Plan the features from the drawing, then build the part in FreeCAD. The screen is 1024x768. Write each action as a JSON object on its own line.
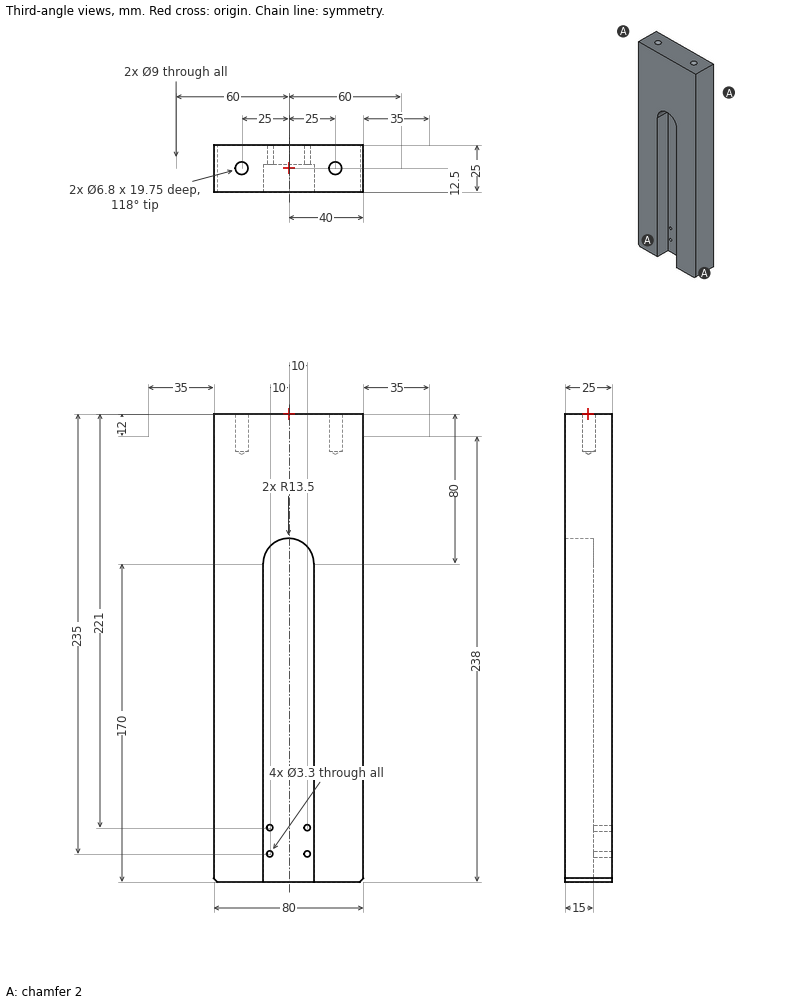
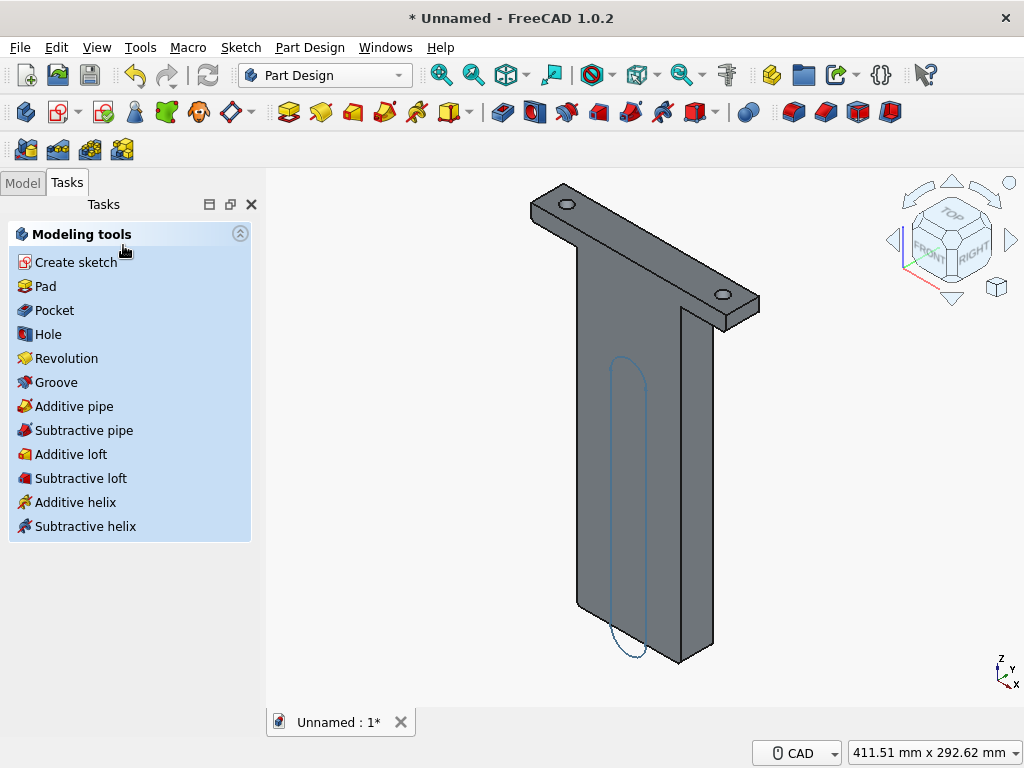
{"action": "left_click", "coordinate": [504, 112]}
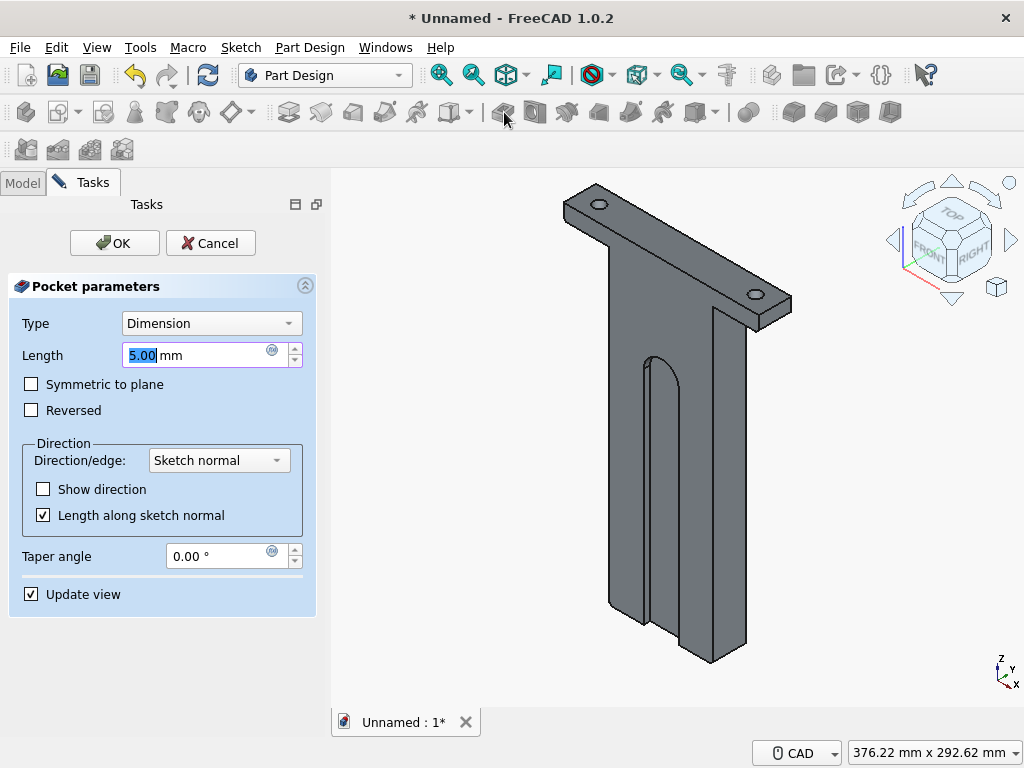
{"action": "type", "text": "15"}
{"action": "key", "text": "Tab"}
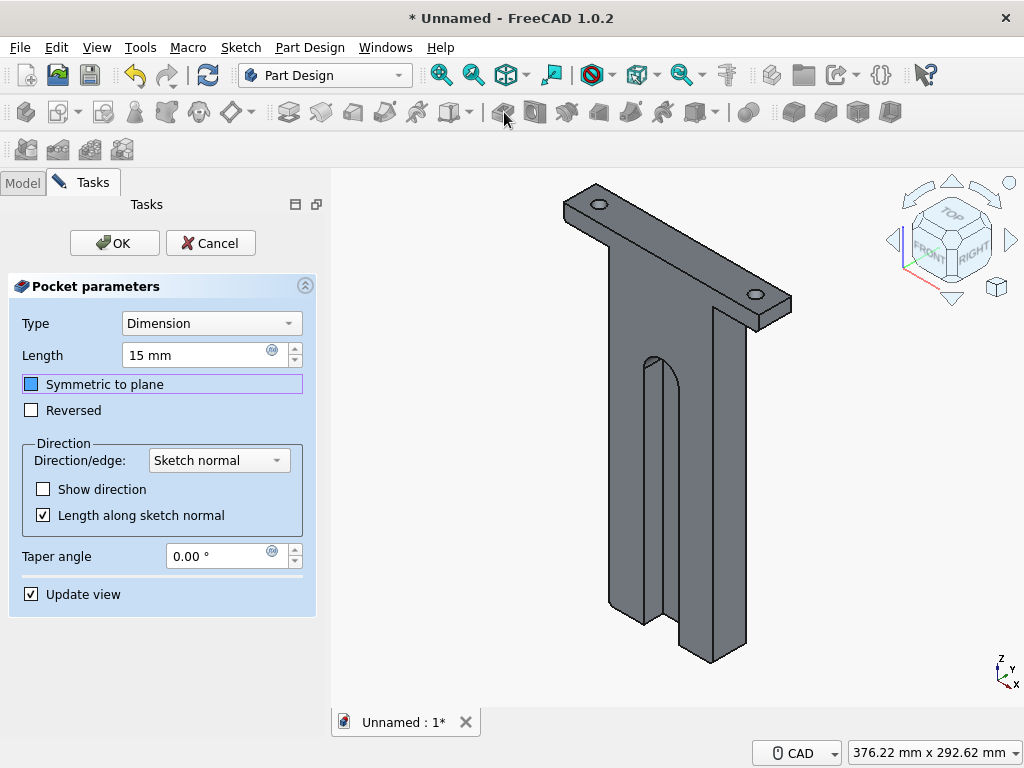
{"action": "left_click", "coordinate": [115, 243]}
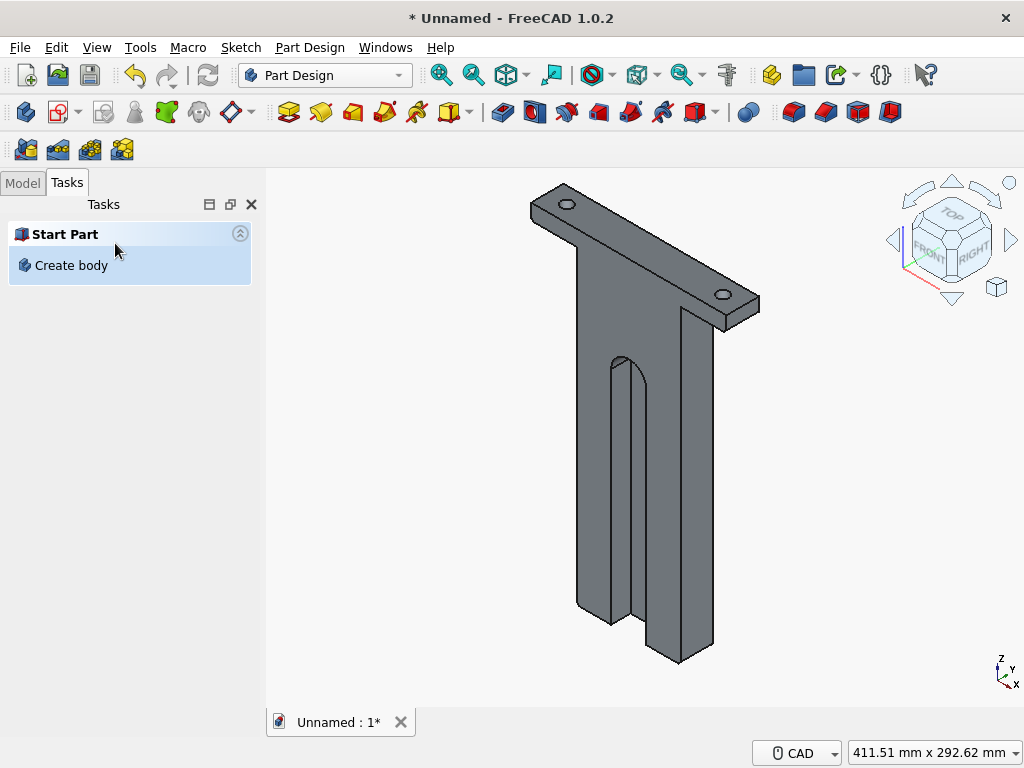
{"action": "key", "text": "4"}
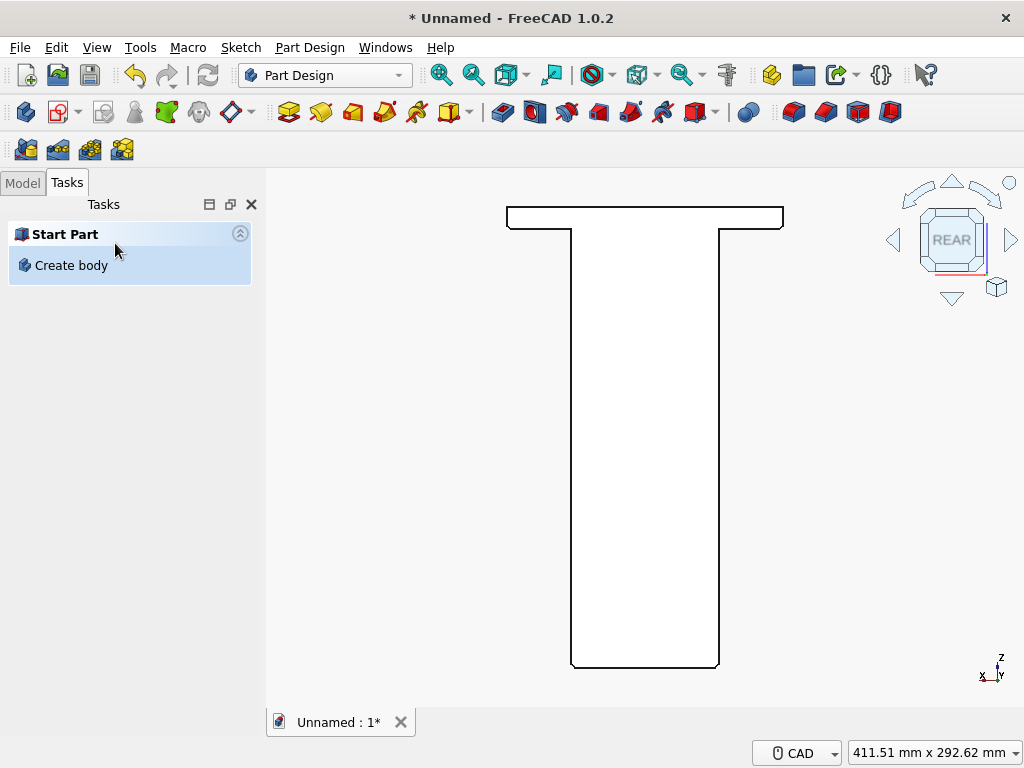
{"action": "left_click", "coordinate": [645, 305]}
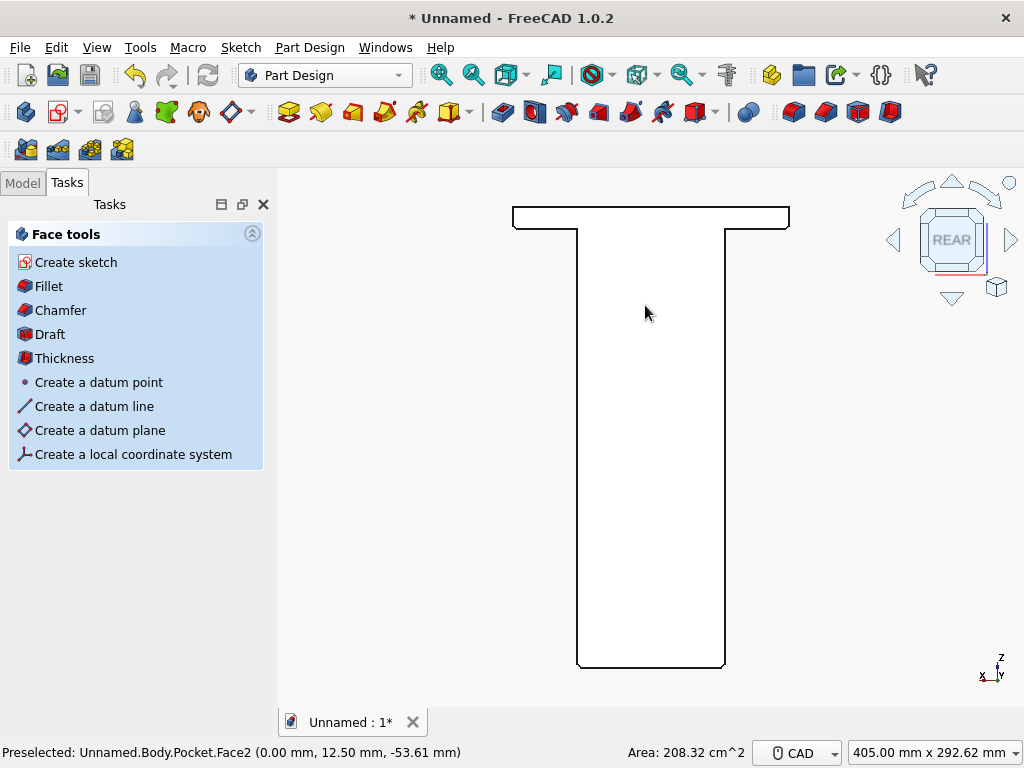
{"action": "left_click", "coordinate": [58, 112]}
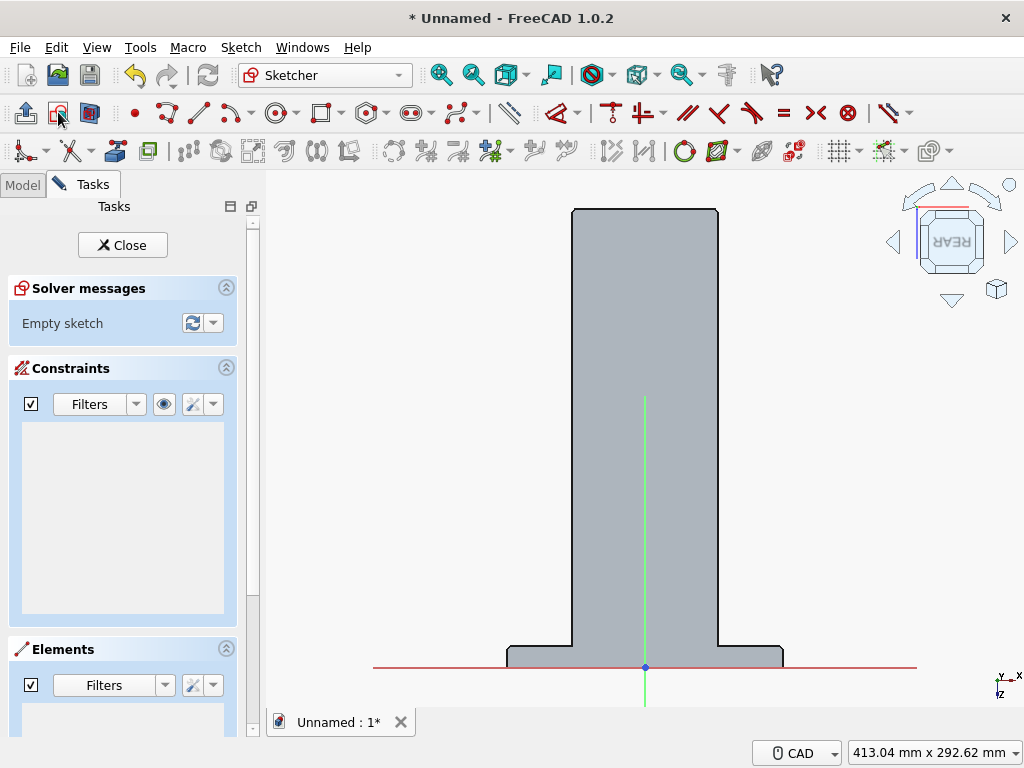
{"action": "scroll", "coordinate": [654, 226], "scroll_direction": "up", "scroll_amount": 11}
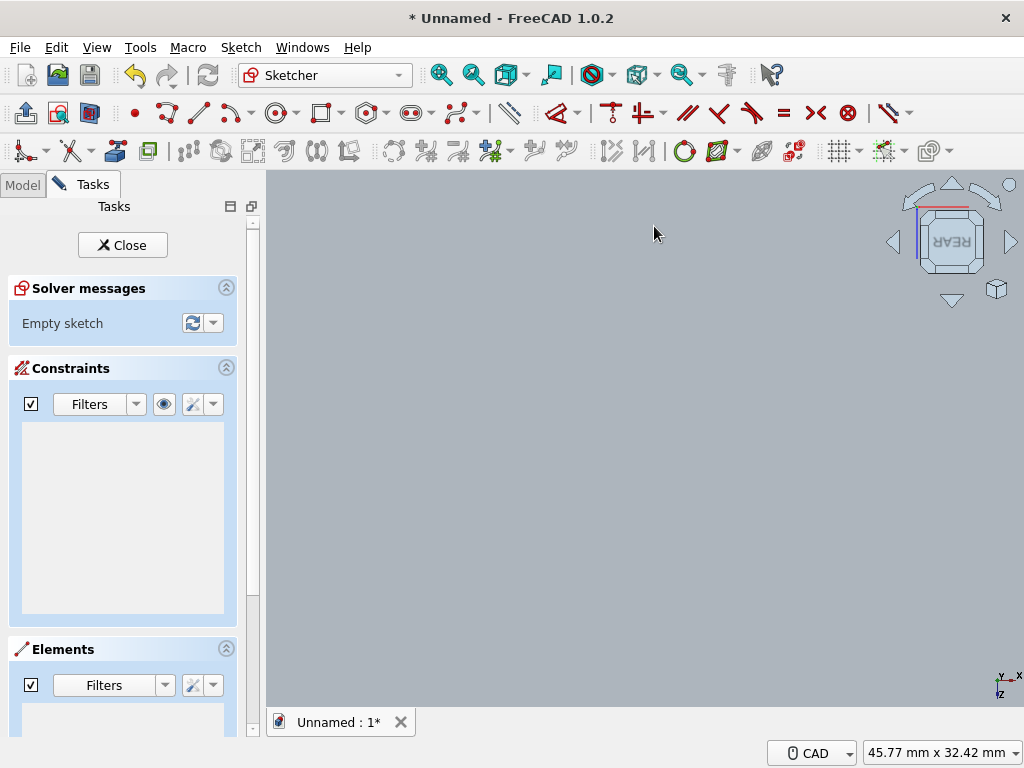
{"action": "left_click", "coordinate": [276, 114]}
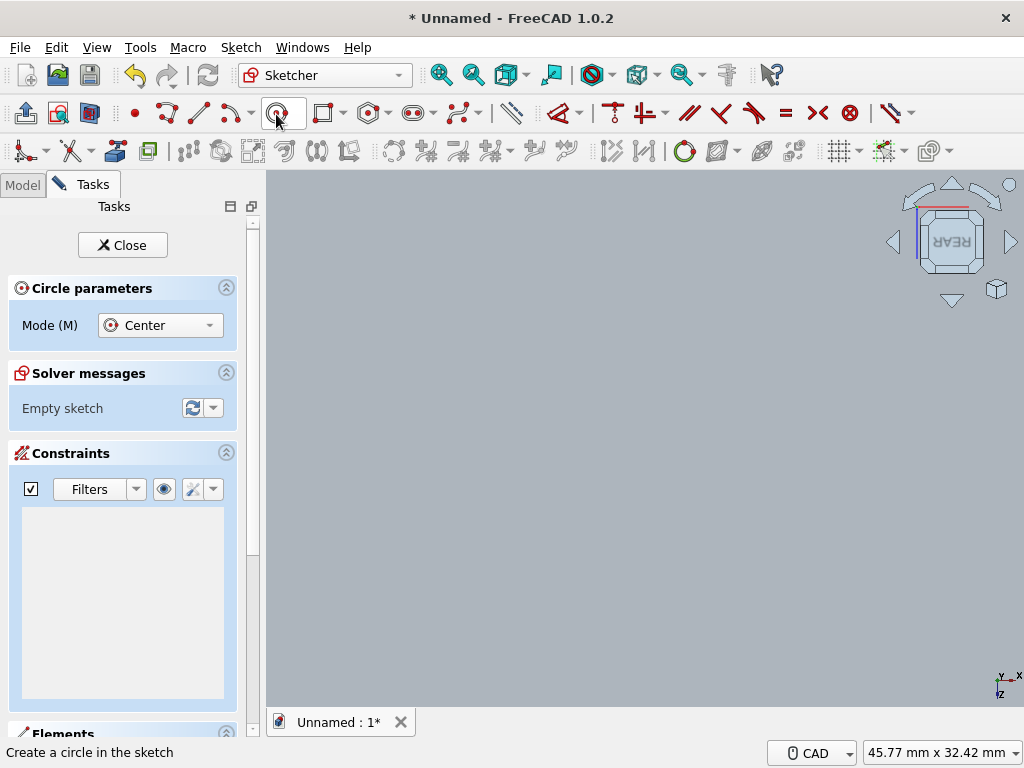
{"action": "left_click", "coordinate": [403, 321]}
{"action": "left_click", "coordinate": [422, 302]}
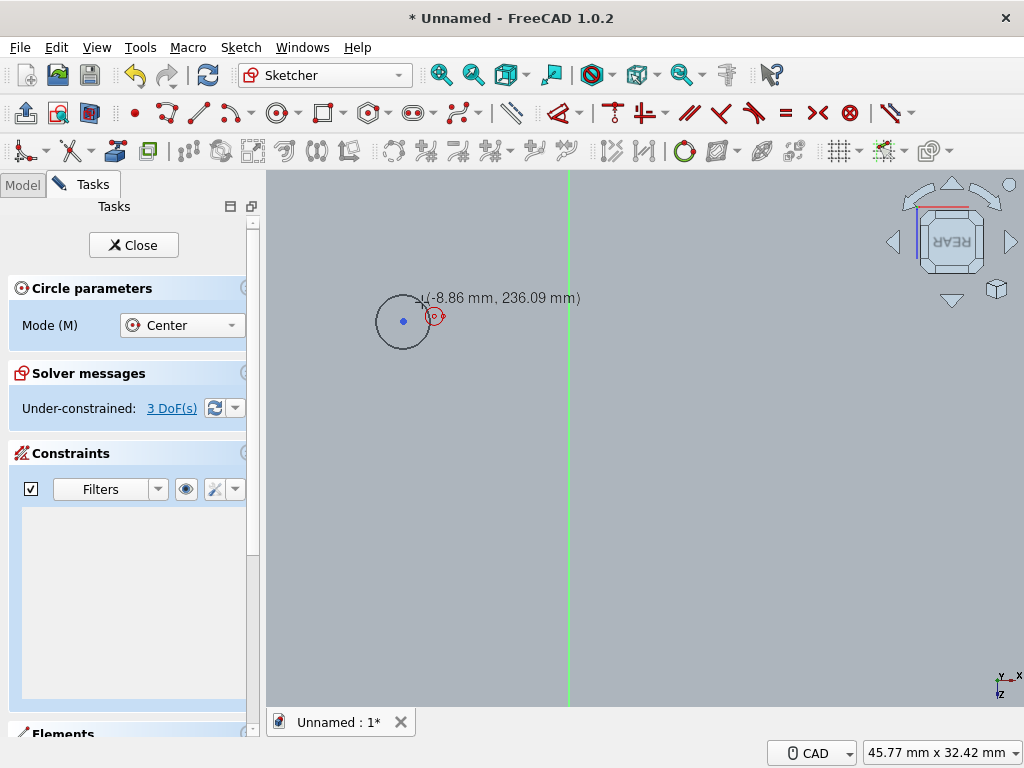
{"action": "left_click", "coordinate": [403, 553]}
{"action": "left_click", "coordinate": [422, 534]}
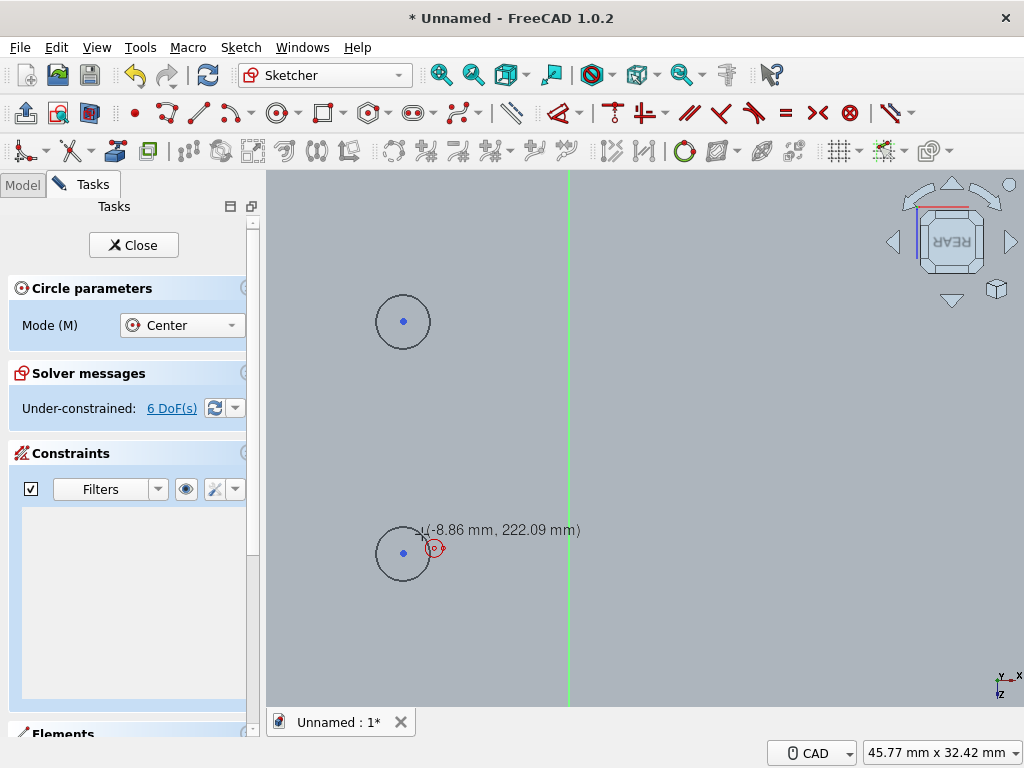
{"action": "left_click", "coordinate": [734, 553]}
{"action": "left_click", "coordinate": [754, 534]}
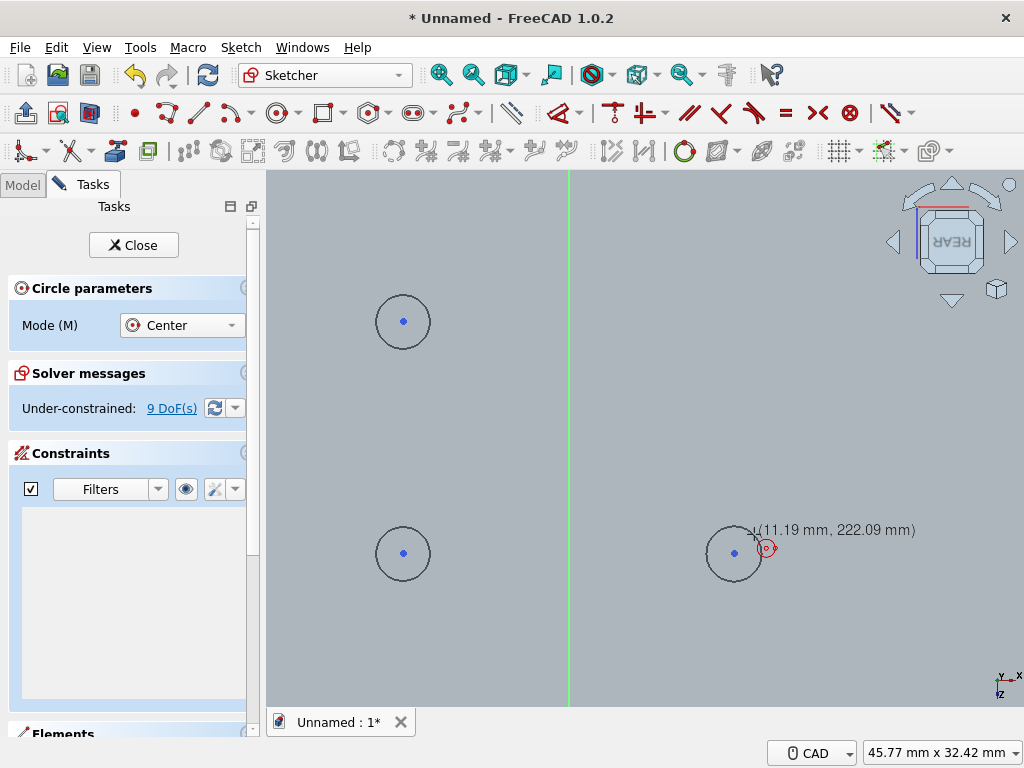
{"action": "left_click", "coordinate": [734, 321]}
{"action": "left_click", "coordinate": [754, 302]}
{"action": "key", "text": "Escape"}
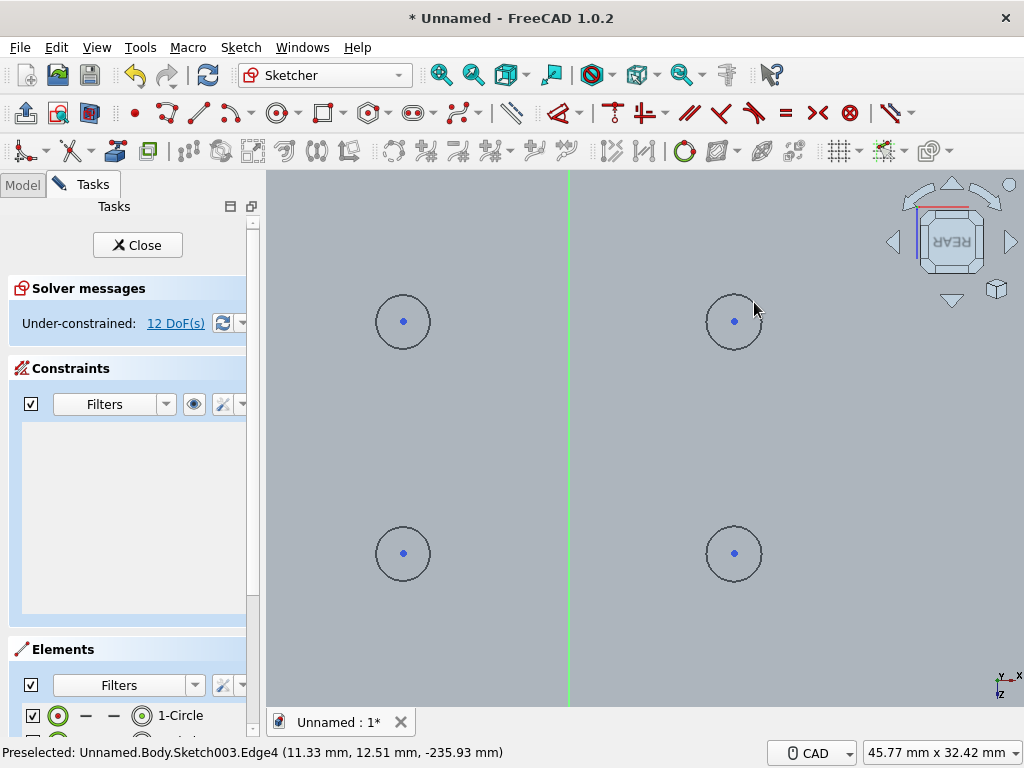
{"action": "left_click", "coordinate": [422, 303]}